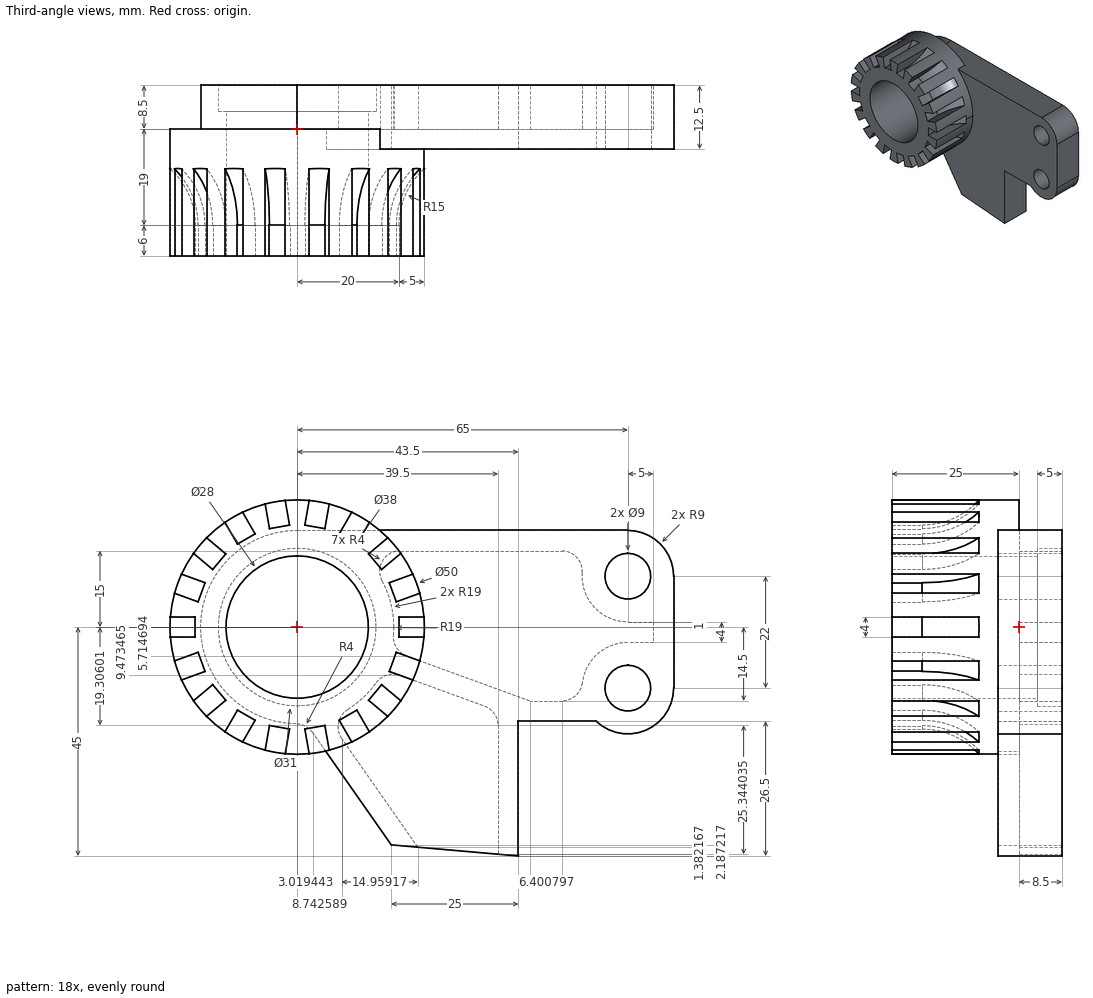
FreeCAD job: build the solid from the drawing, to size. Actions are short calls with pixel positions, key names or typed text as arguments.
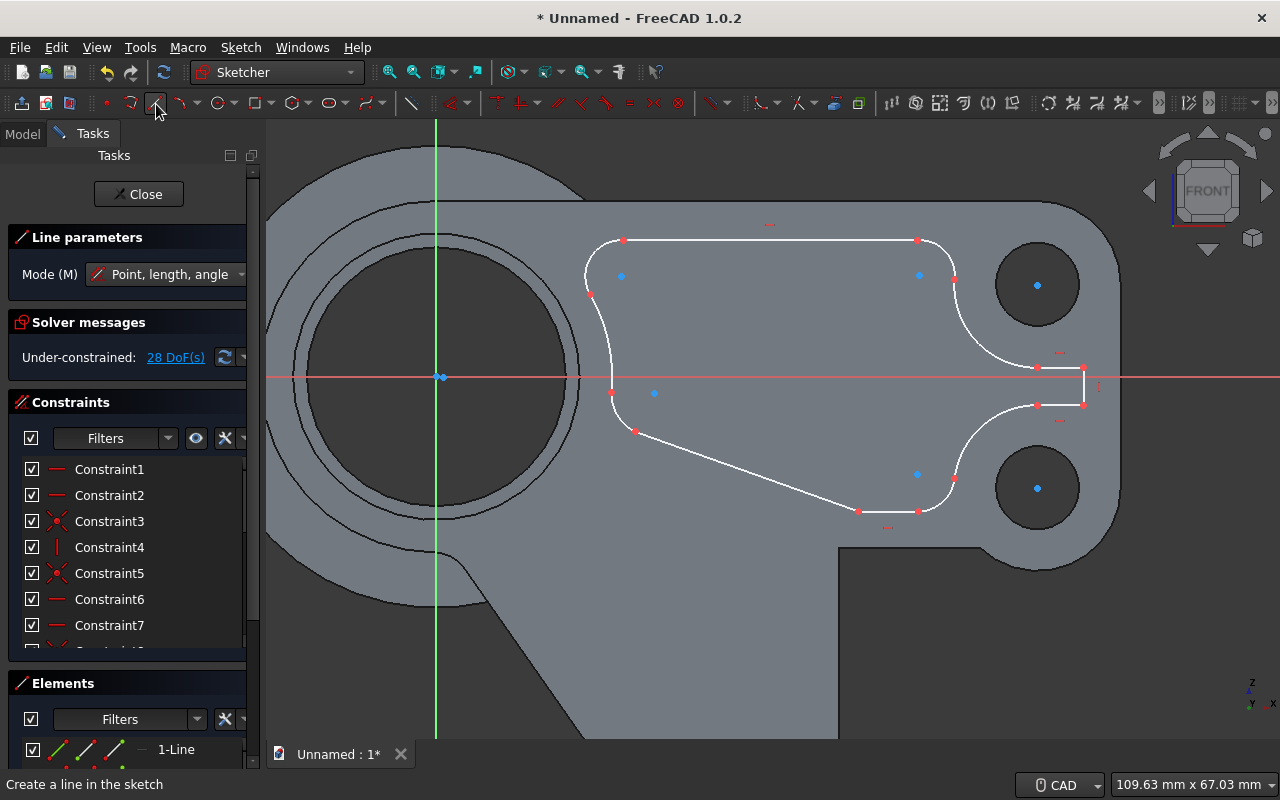
click(623, 464)
click(777, 521)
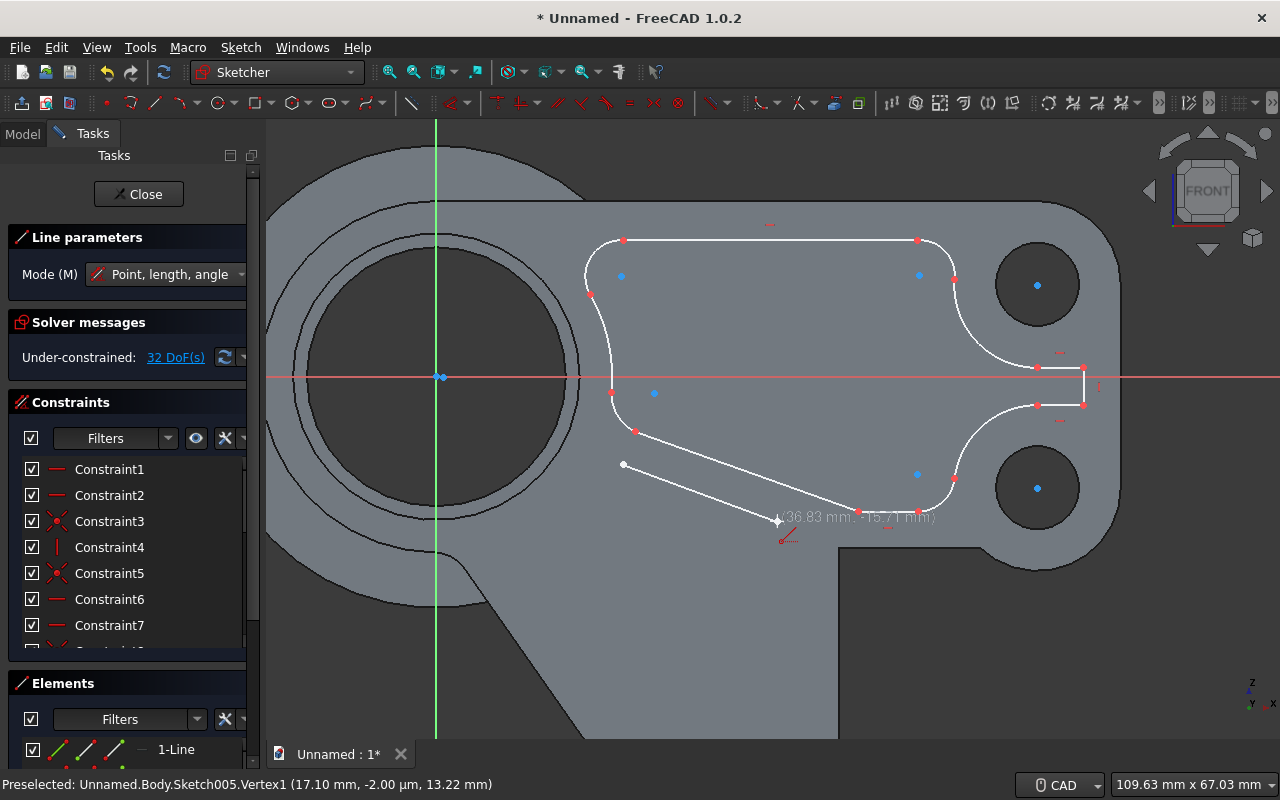
click(132, 104)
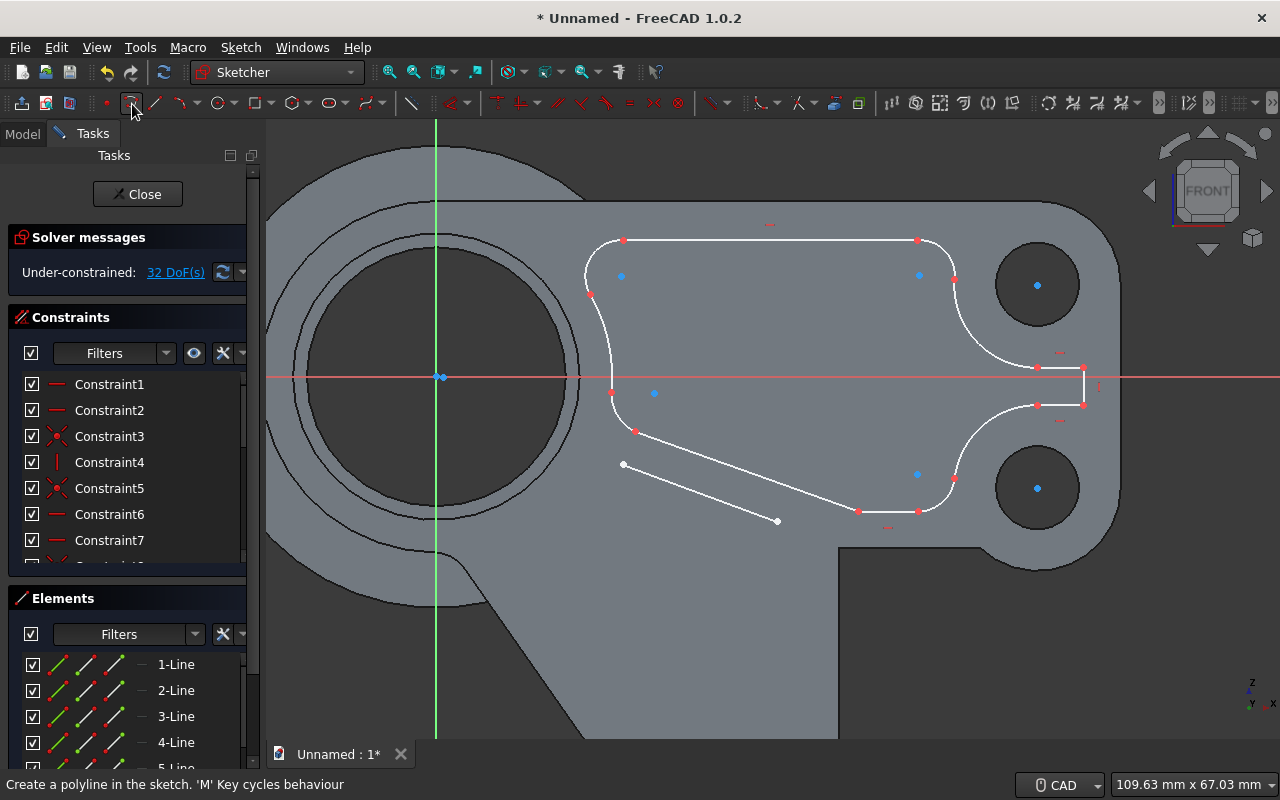
click(802, 555)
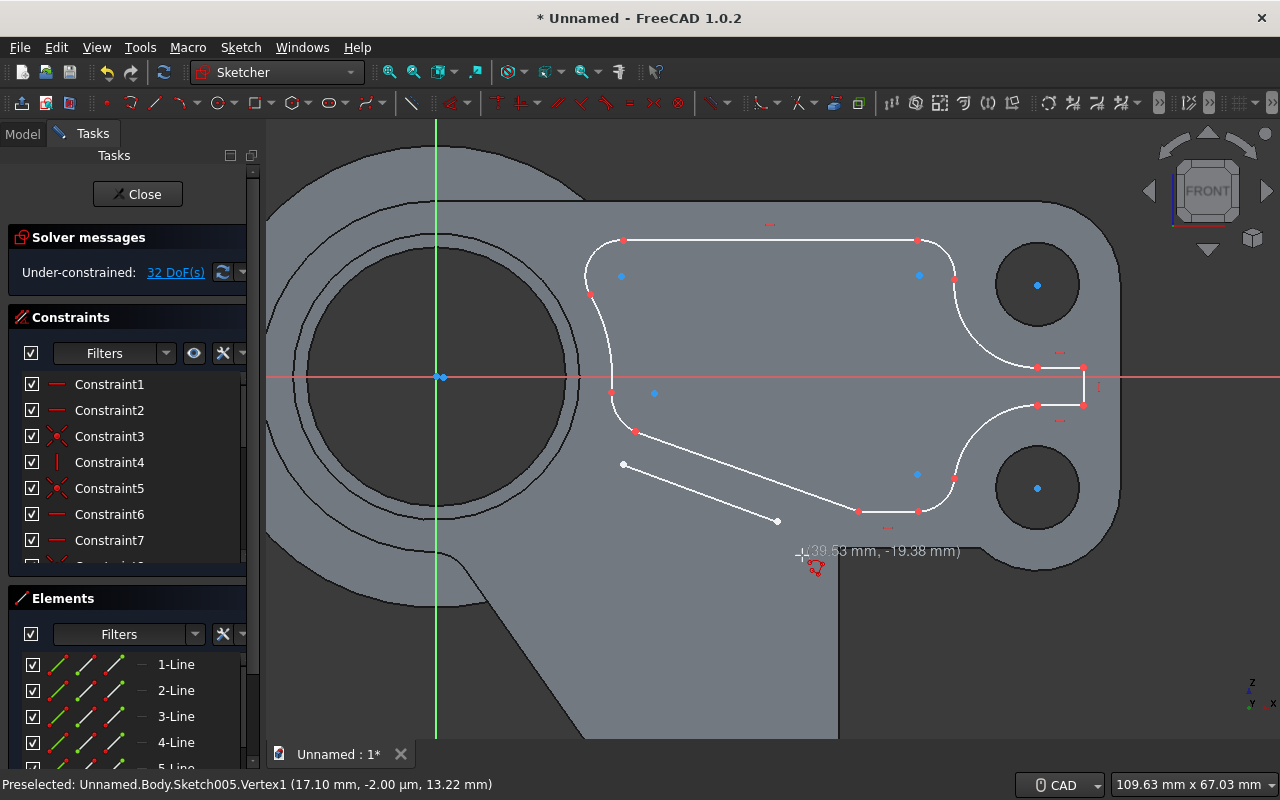
scroll(592, 257, down, 2)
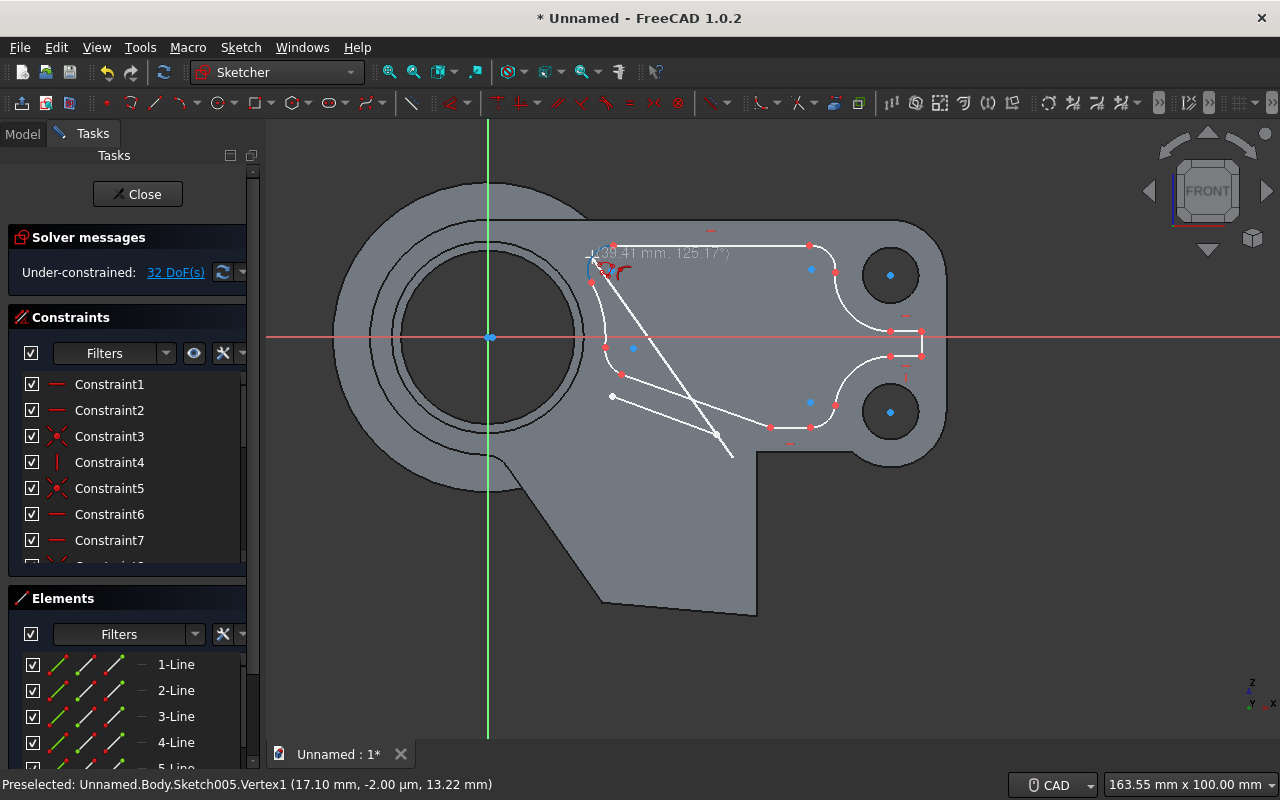
click(733, 614)
click(635, 606)
click(542, 473)
right_click(542, 473)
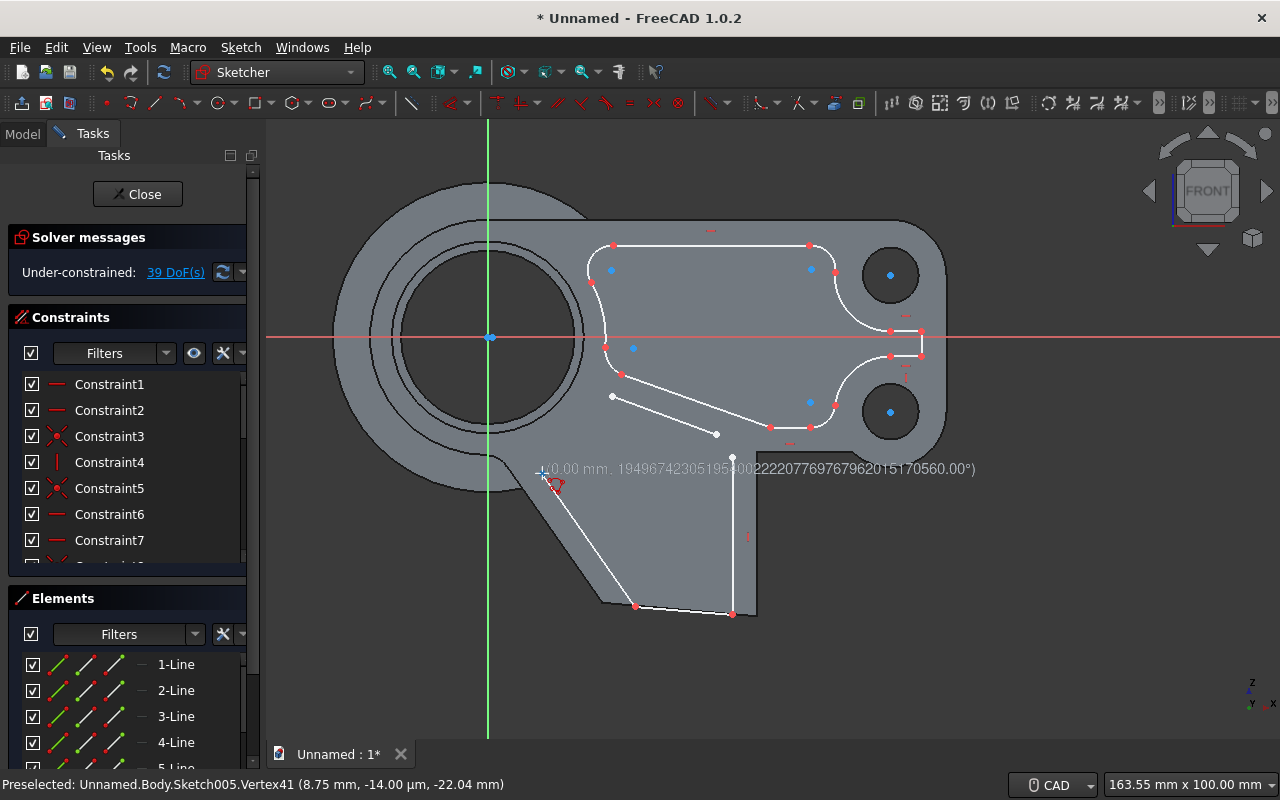
click(180, 104)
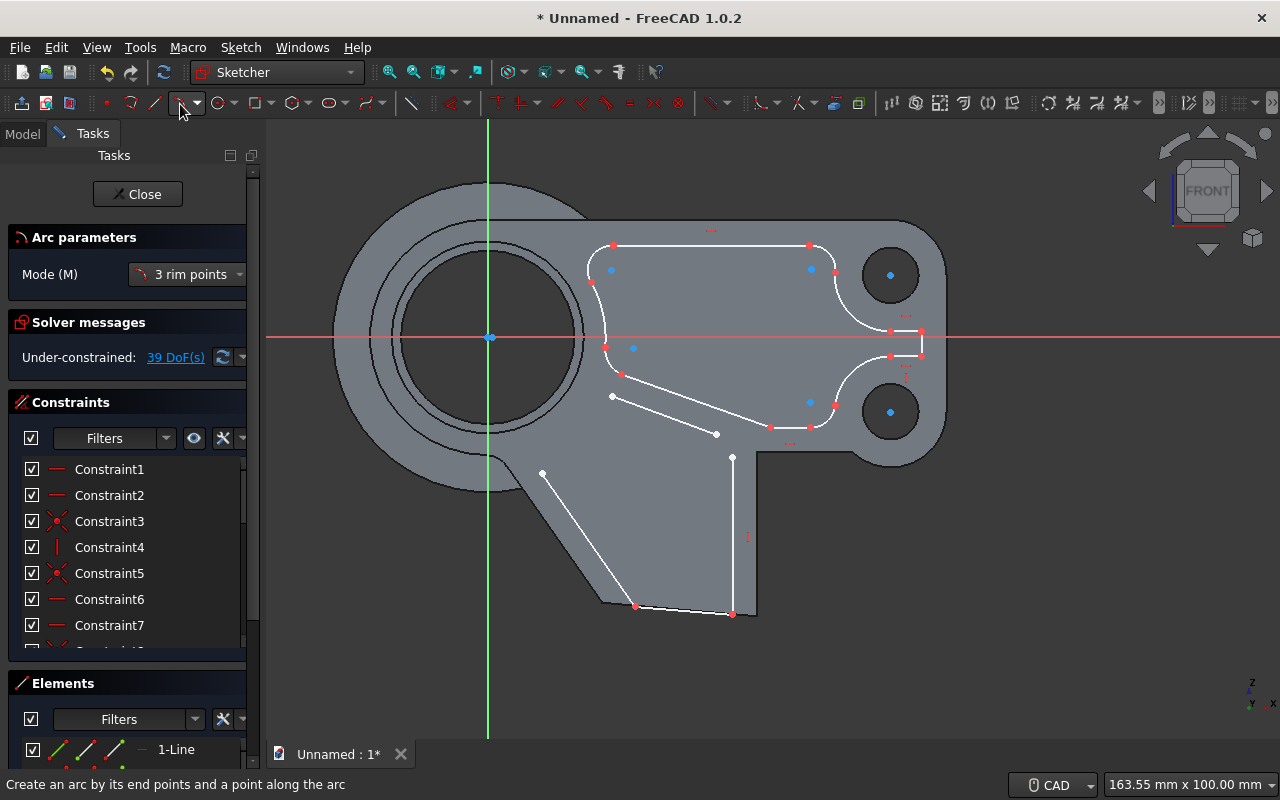
click(716, 435)
click(733, 457)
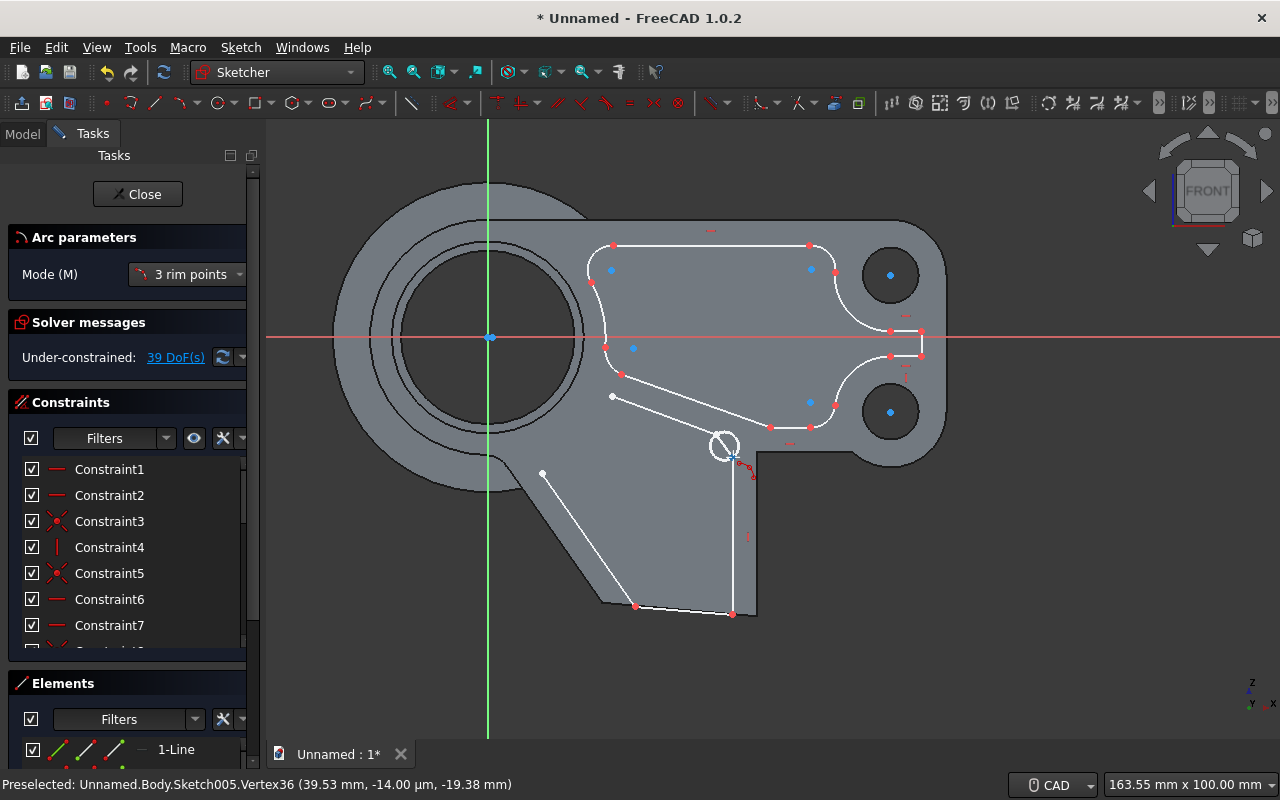
scroll(728, 443, up, 7)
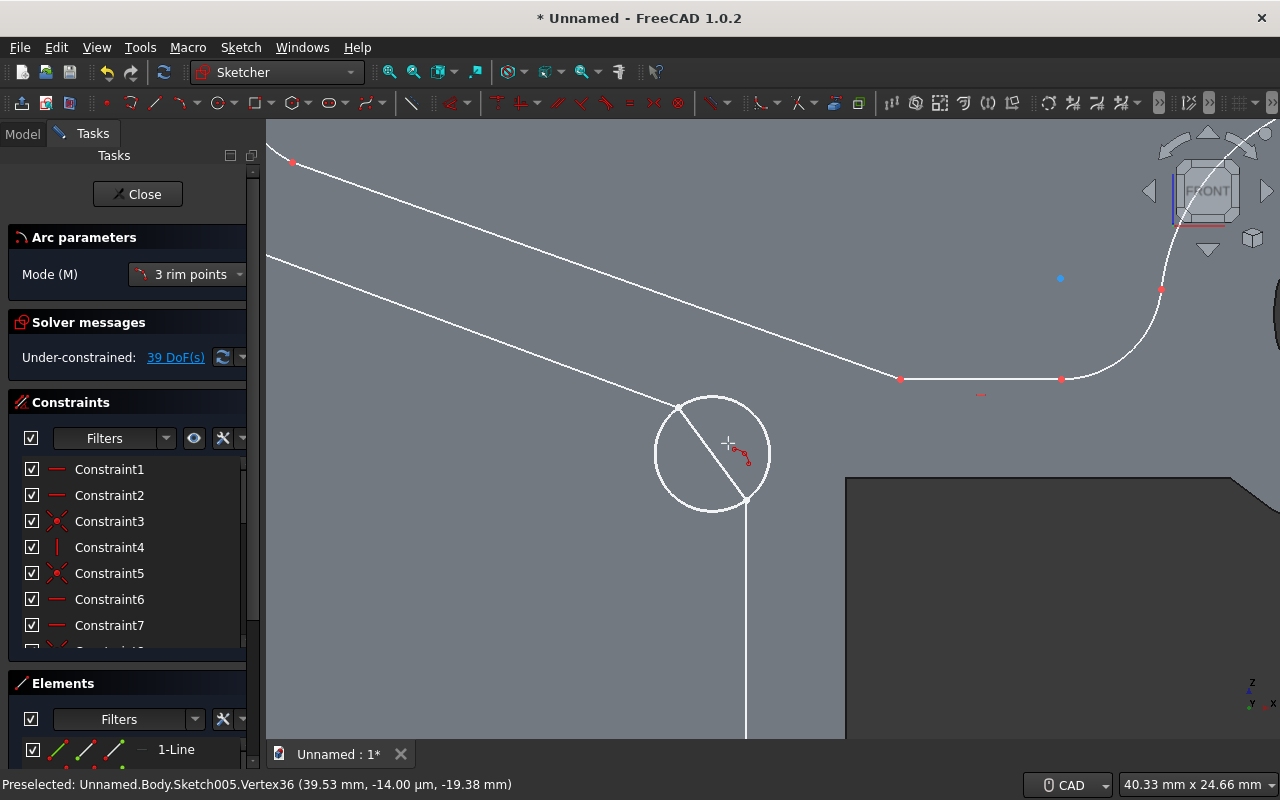
click(727, 441)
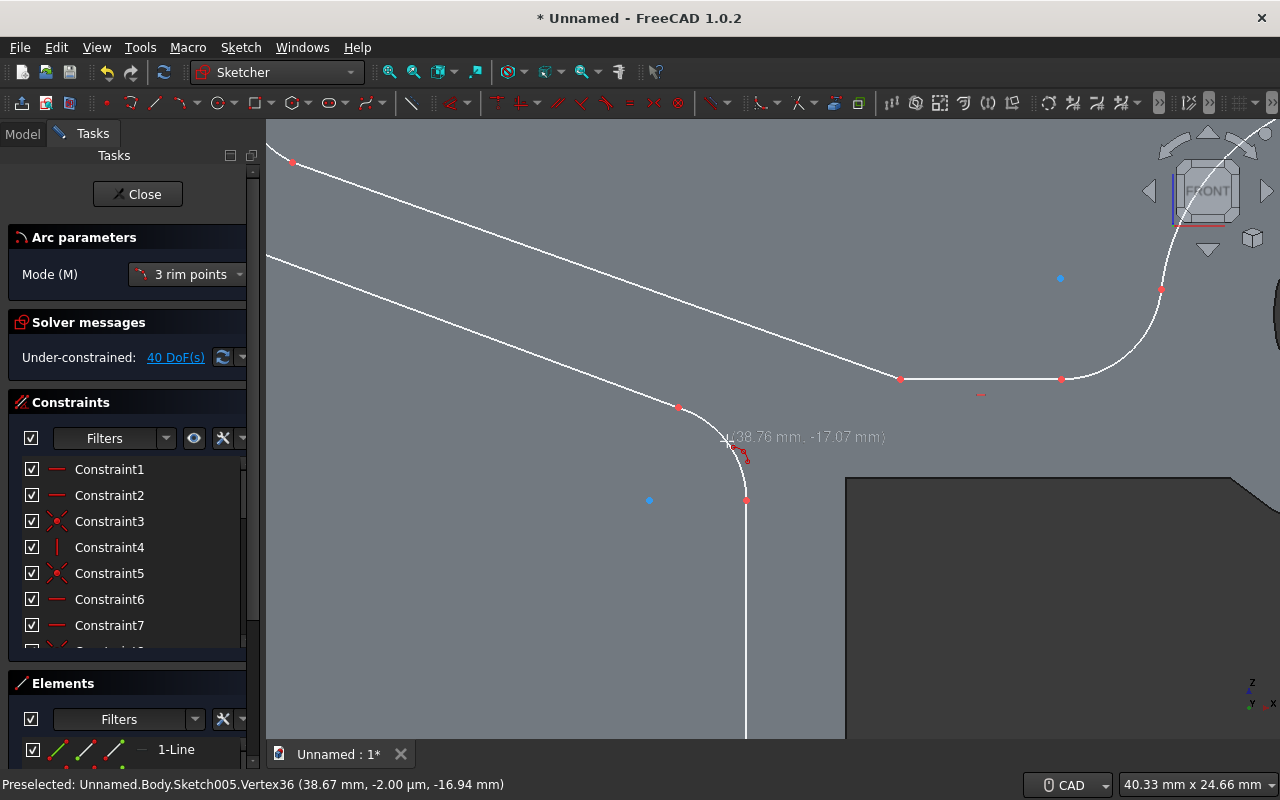
scroll(728, 443, down, 7)